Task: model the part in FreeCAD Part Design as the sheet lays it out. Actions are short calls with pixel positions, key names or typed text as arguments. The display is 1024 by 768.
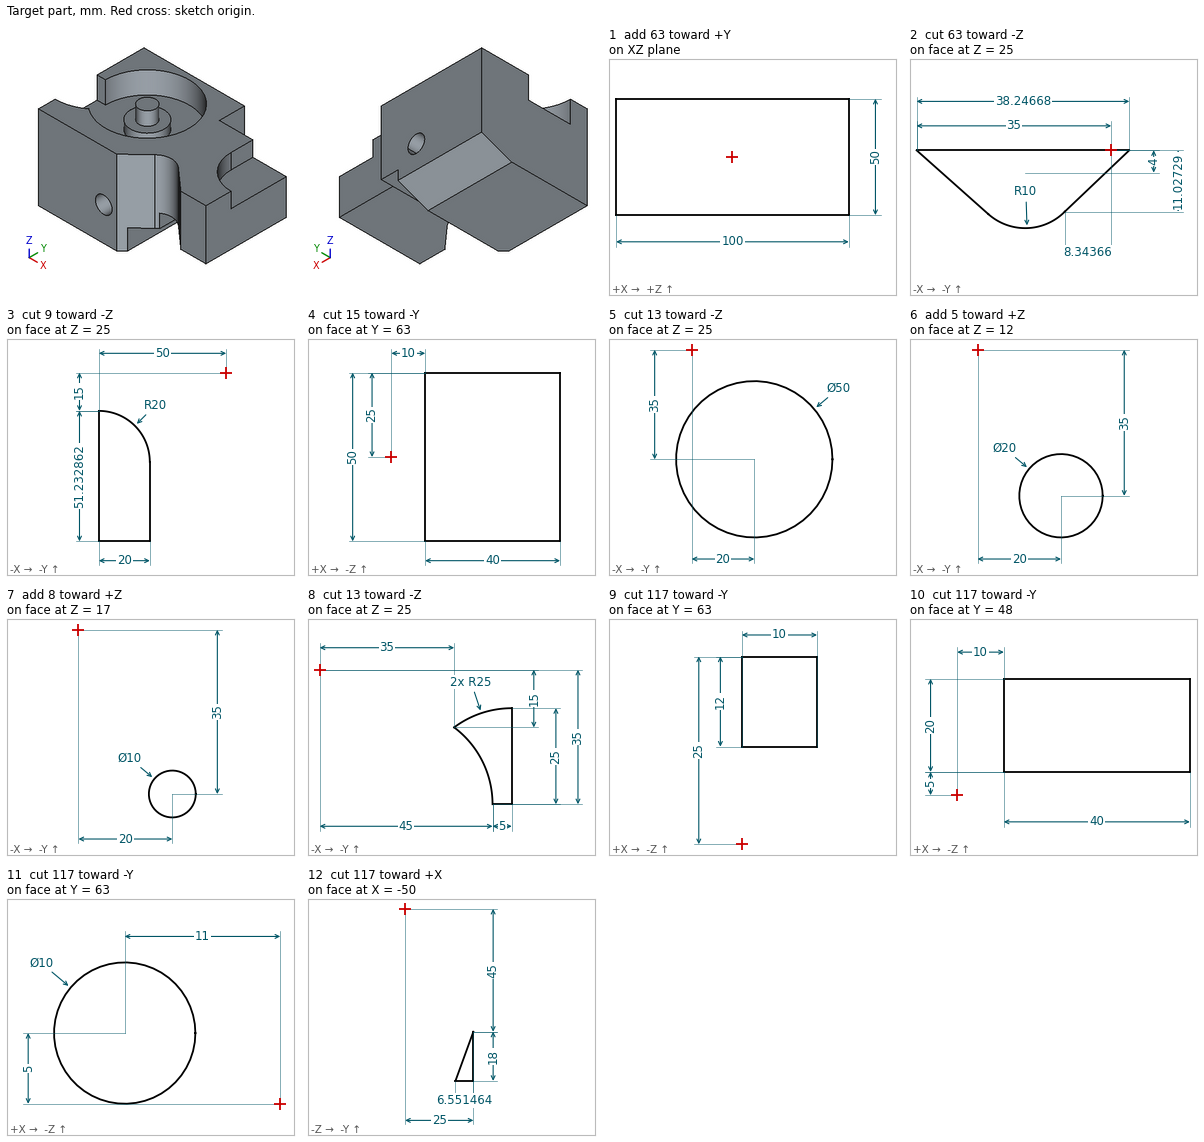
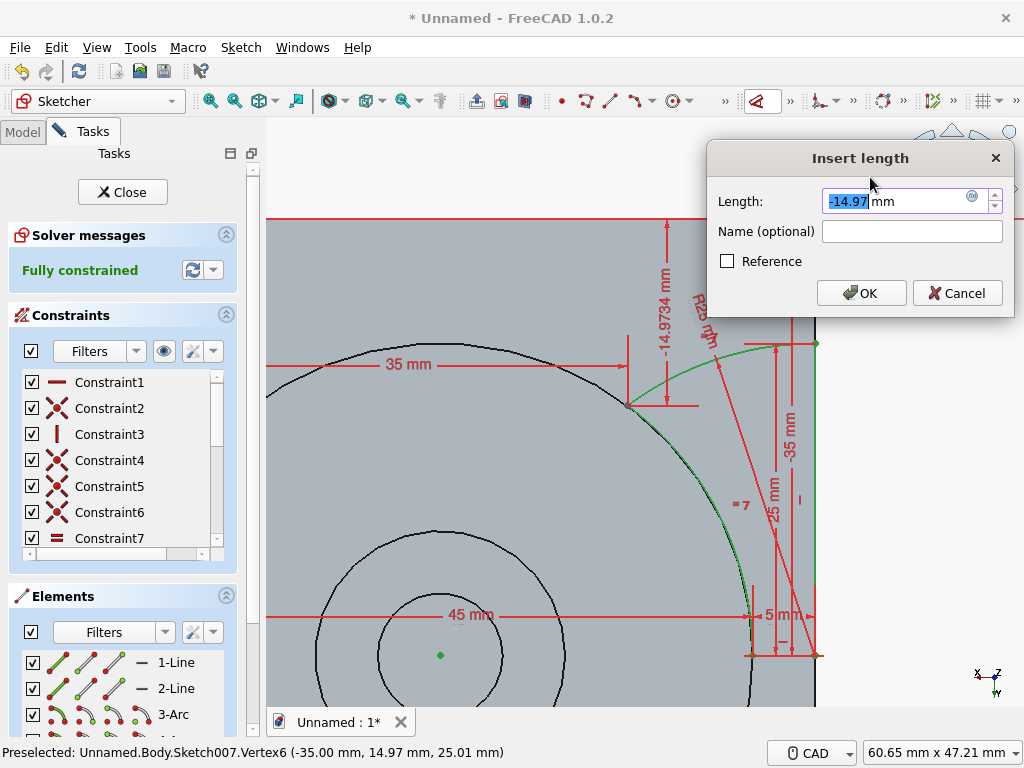
text(-15)
key(Return)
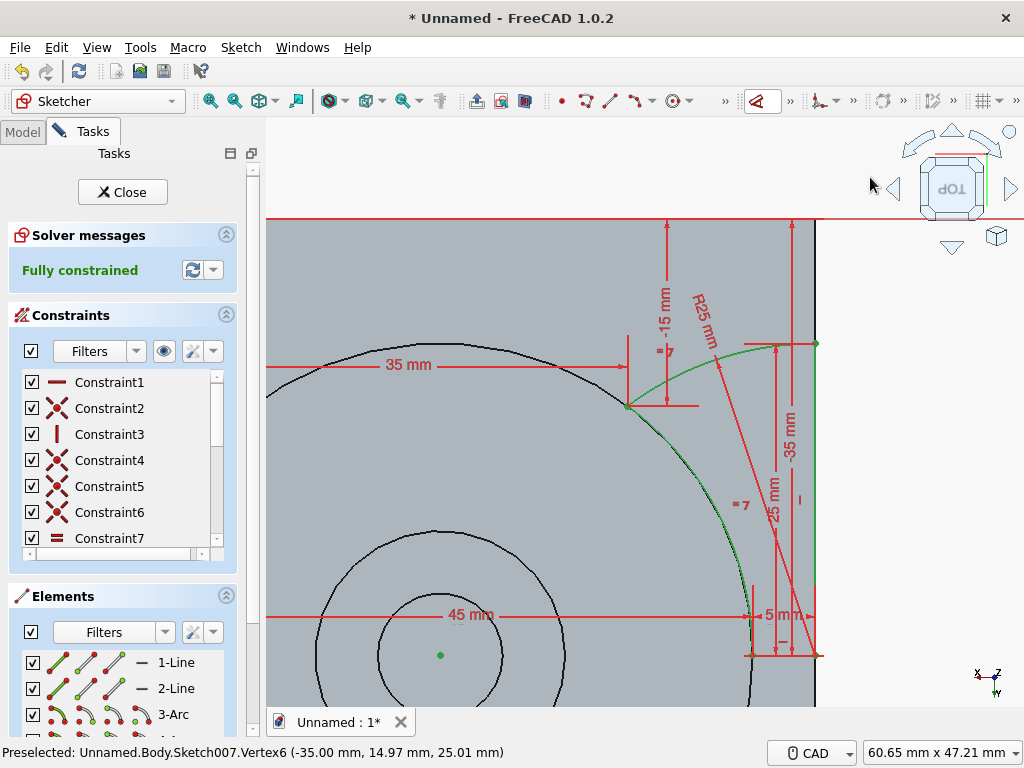
click(123, 192)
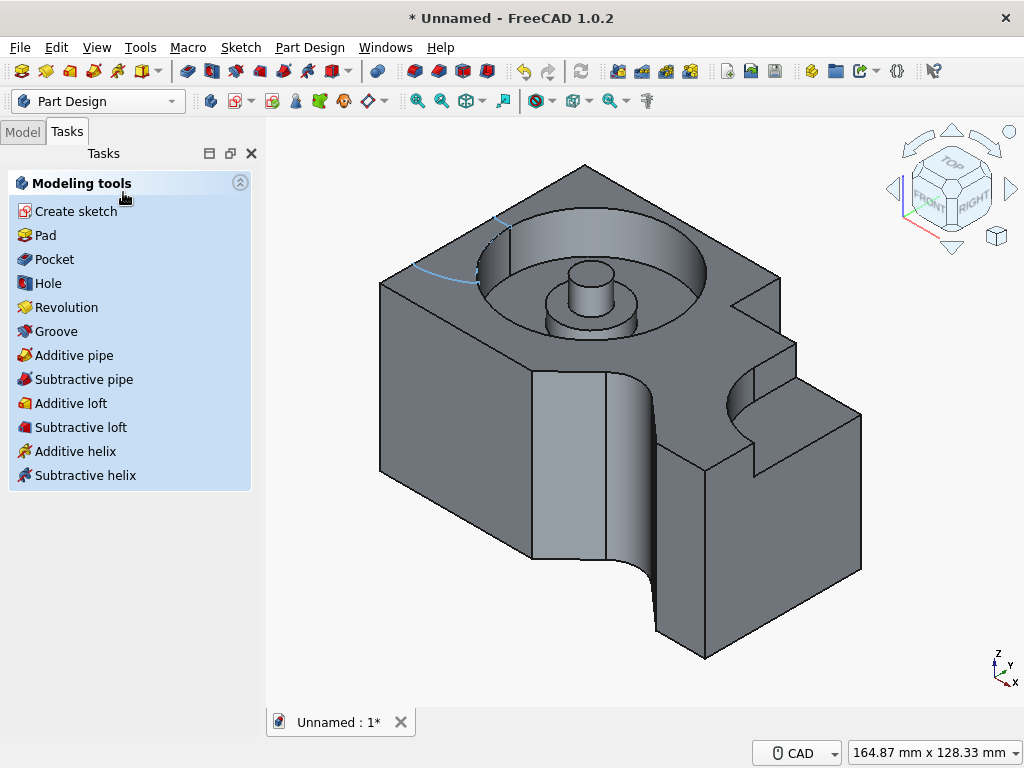
click(188, 72)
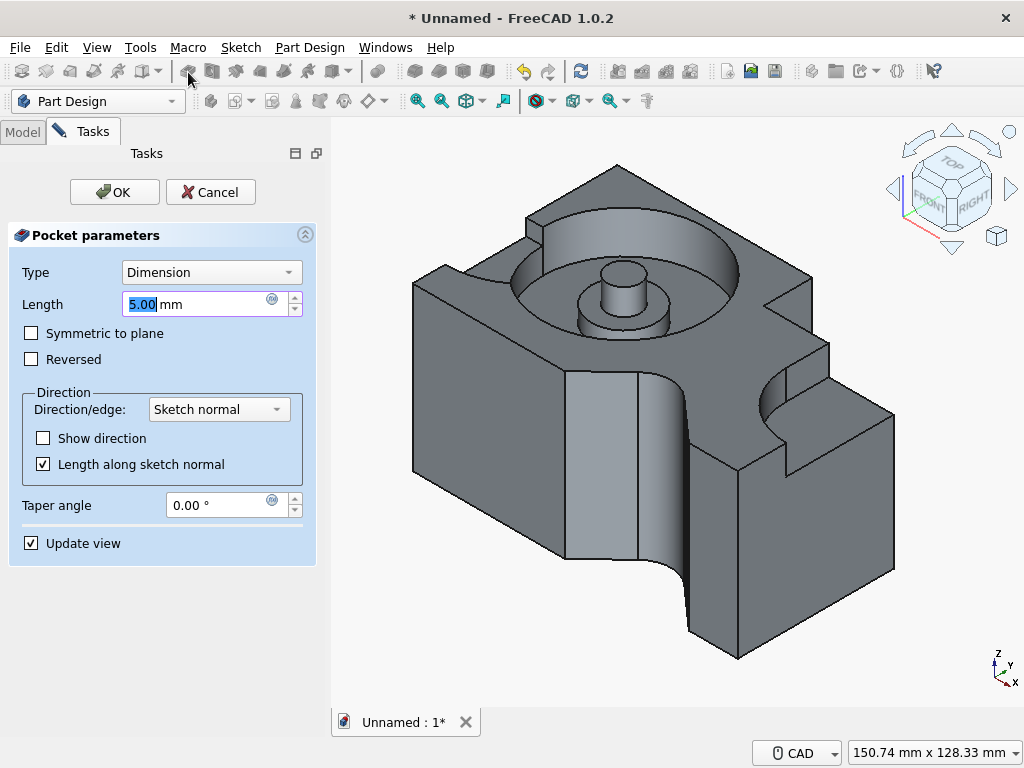
text(13)
key(Tab)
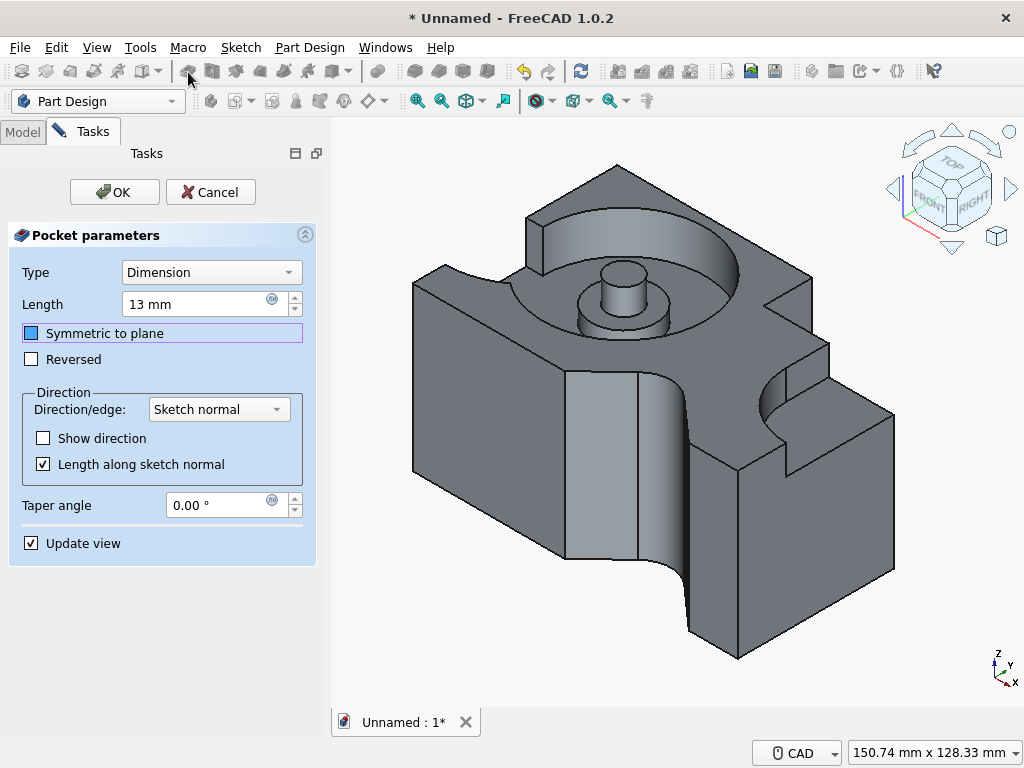
click(115, 192)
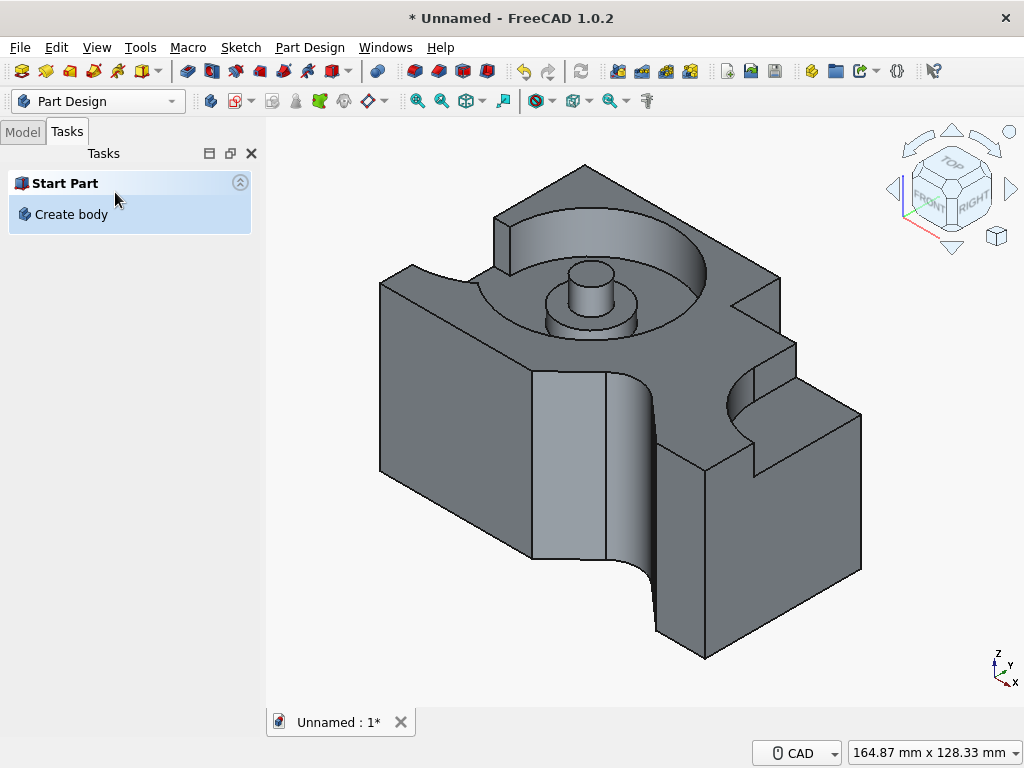
key(4)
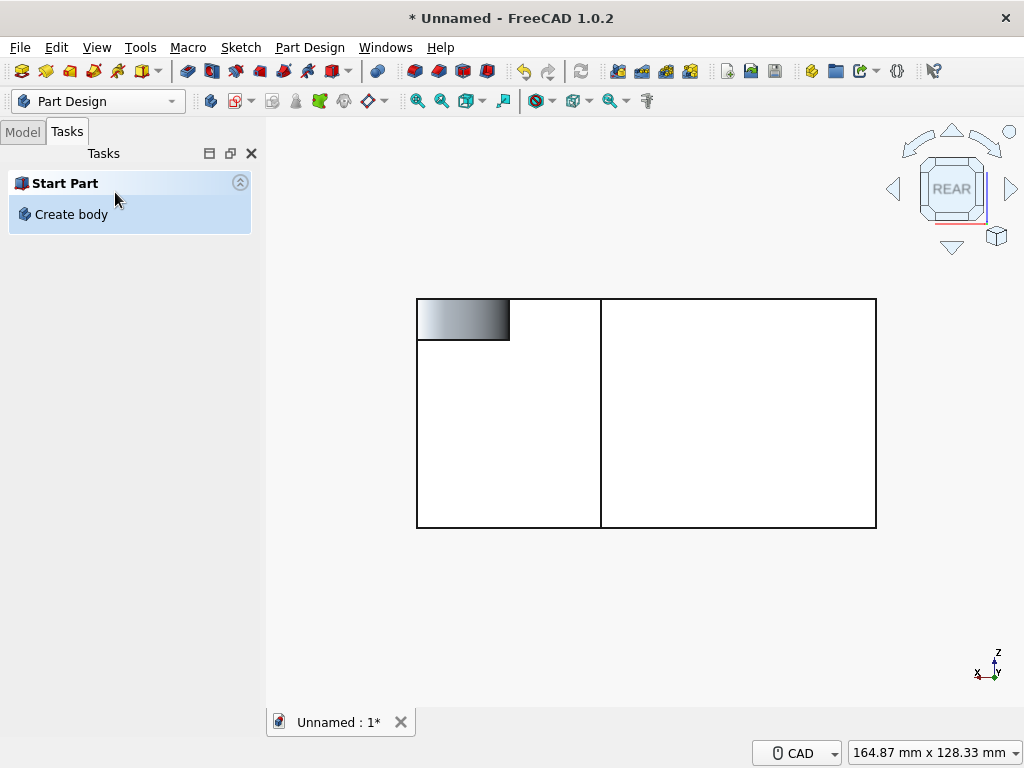
click(738, 412)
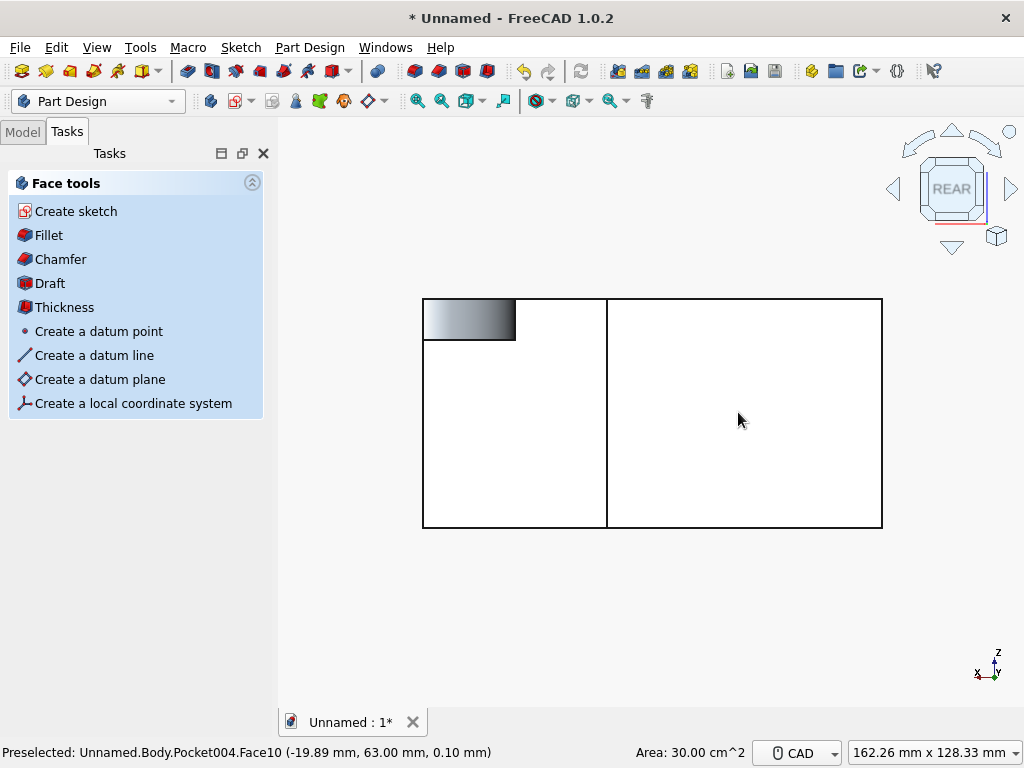
click(236, 102)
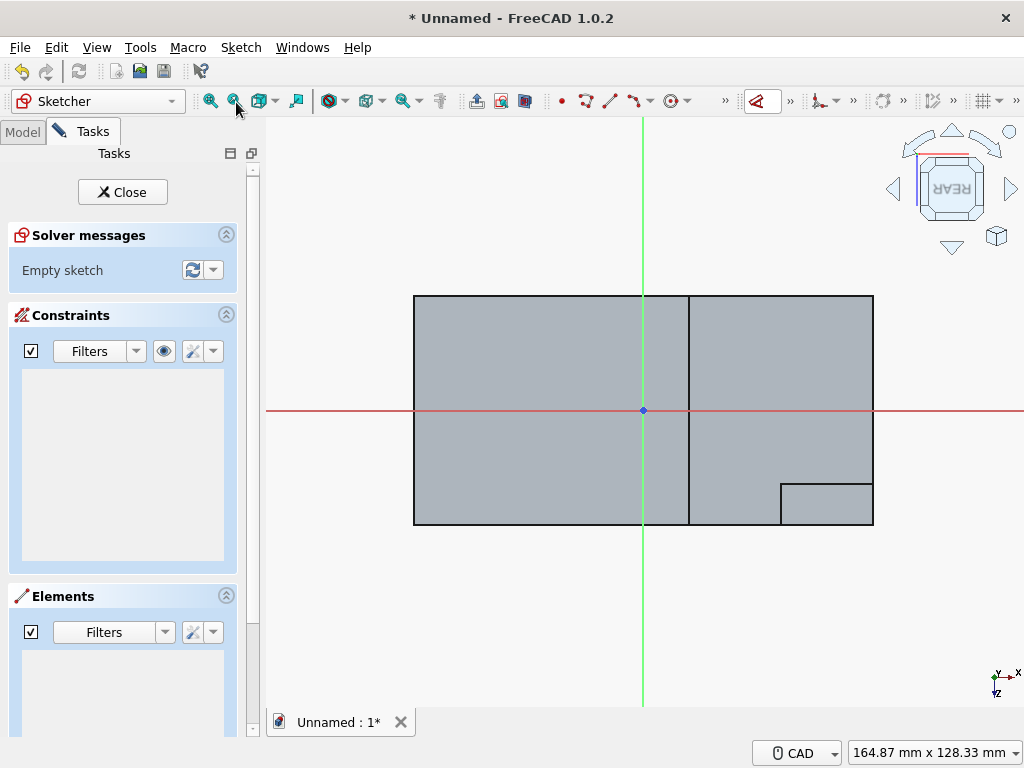
scroll(705, 328, up, 6)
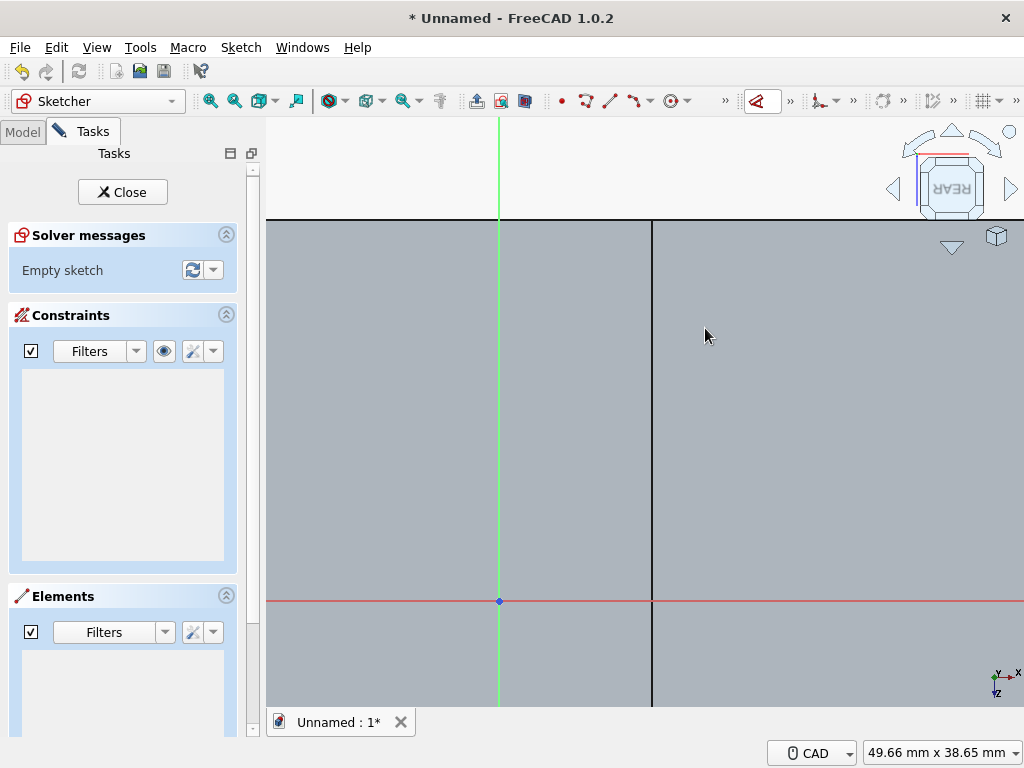
key(g)
key(r)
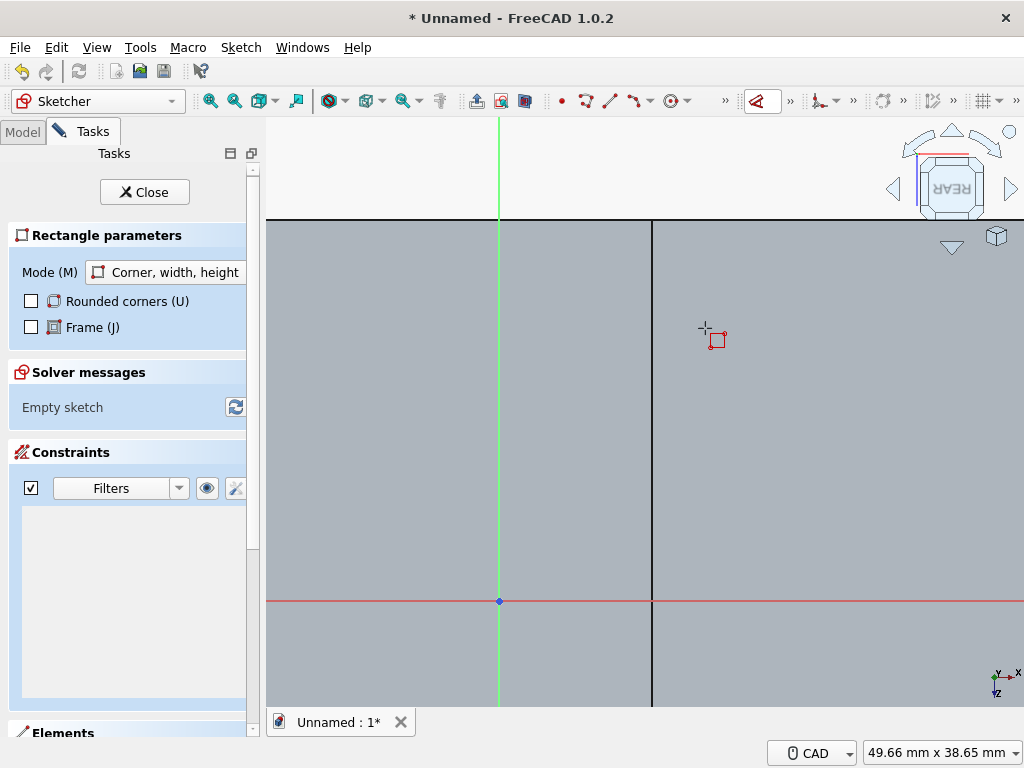
click(499, 220)
click(652, 403)
key(Escape)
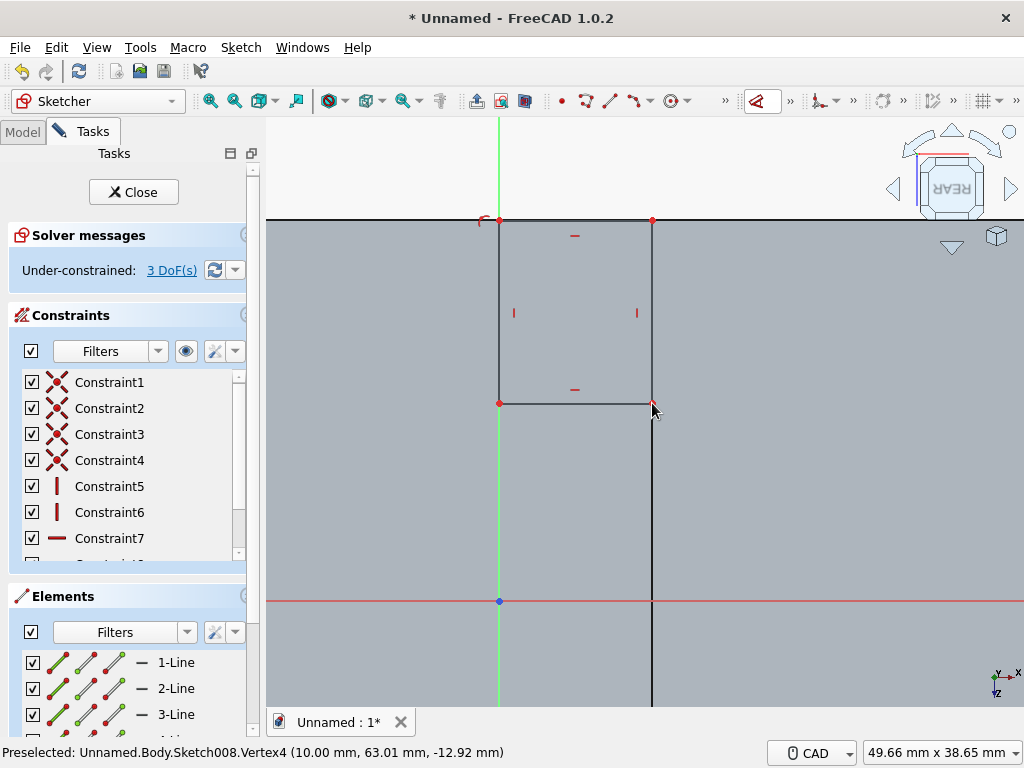
click(499, 276)